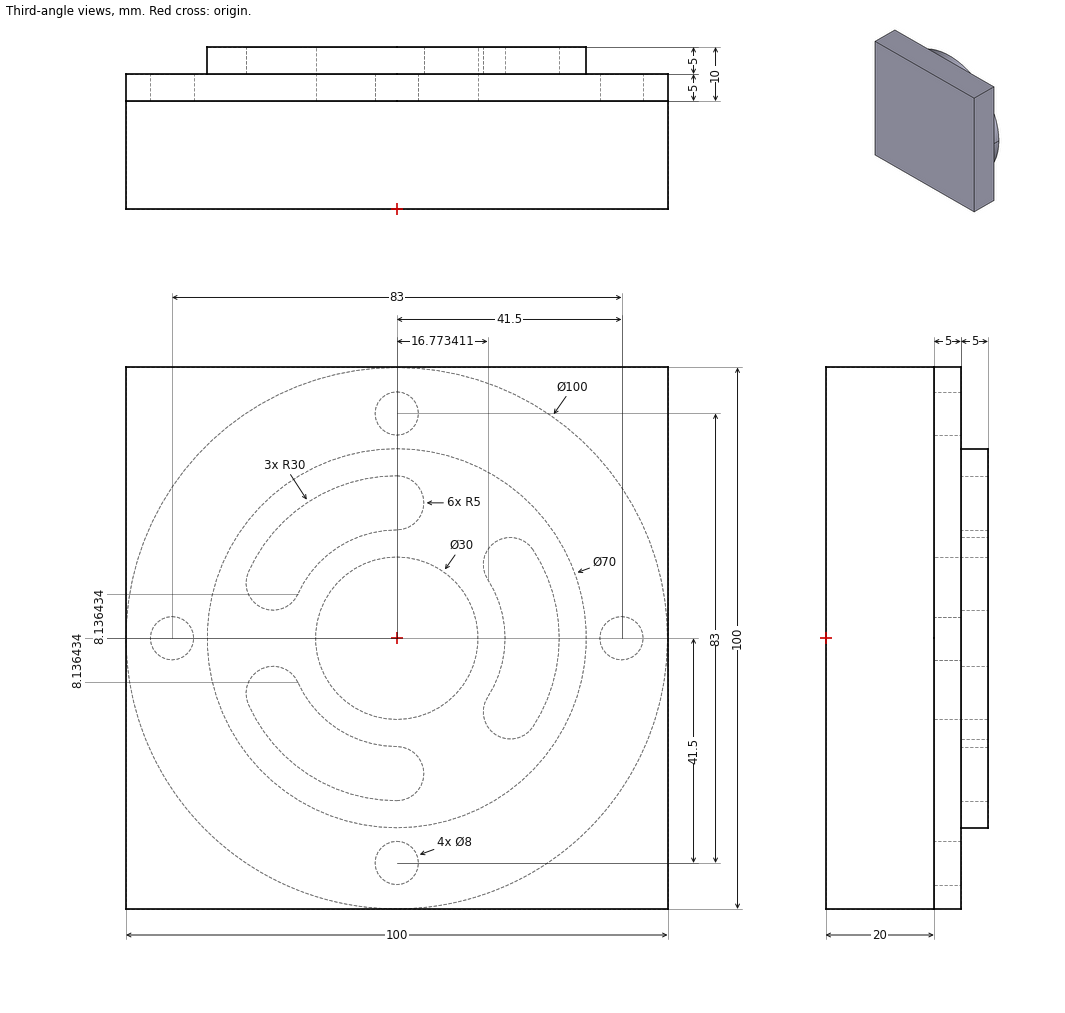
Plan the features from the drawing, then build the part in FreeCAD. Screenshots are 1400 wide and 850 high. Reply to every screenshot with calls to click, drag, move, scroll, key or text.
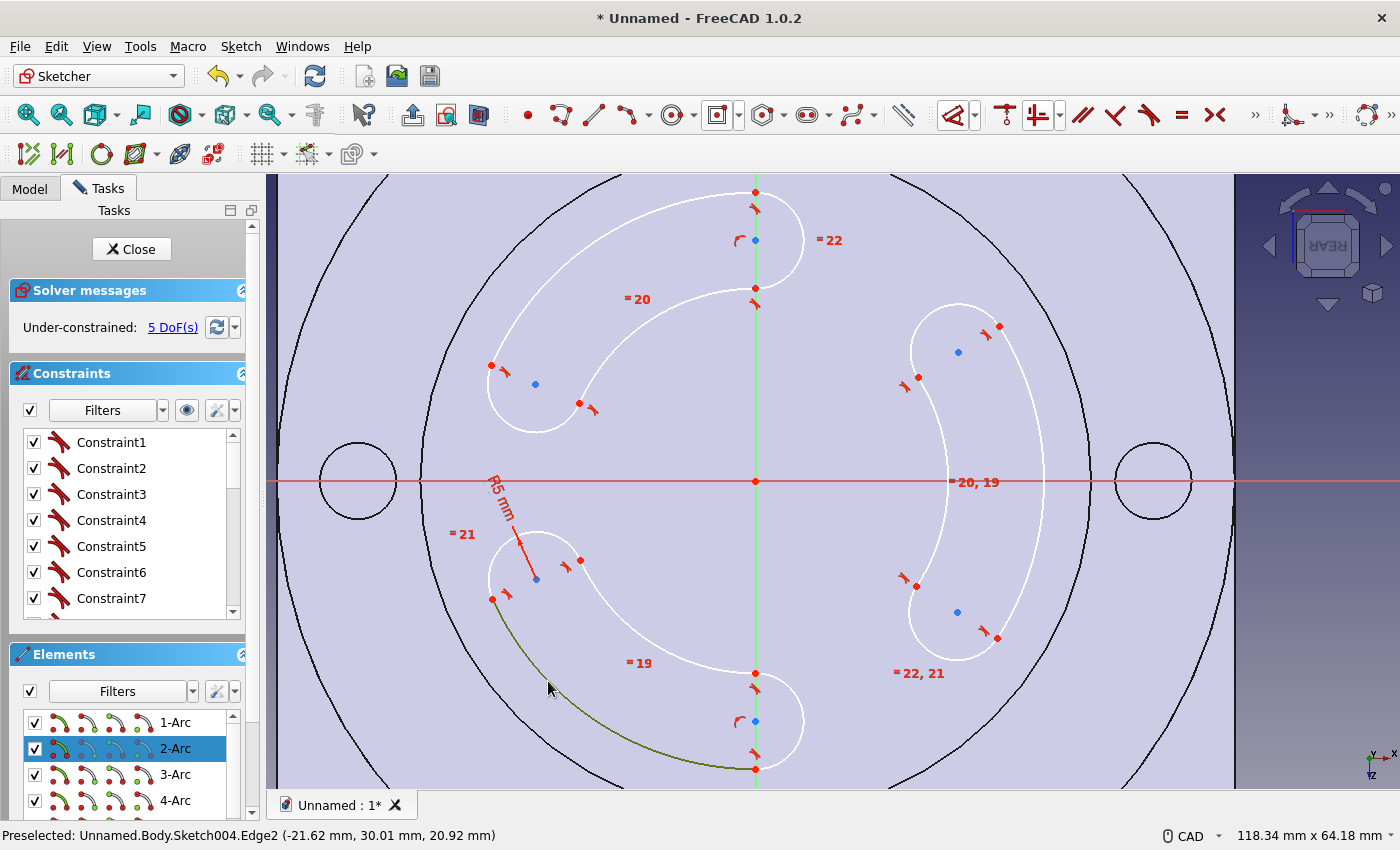
click(974, 116)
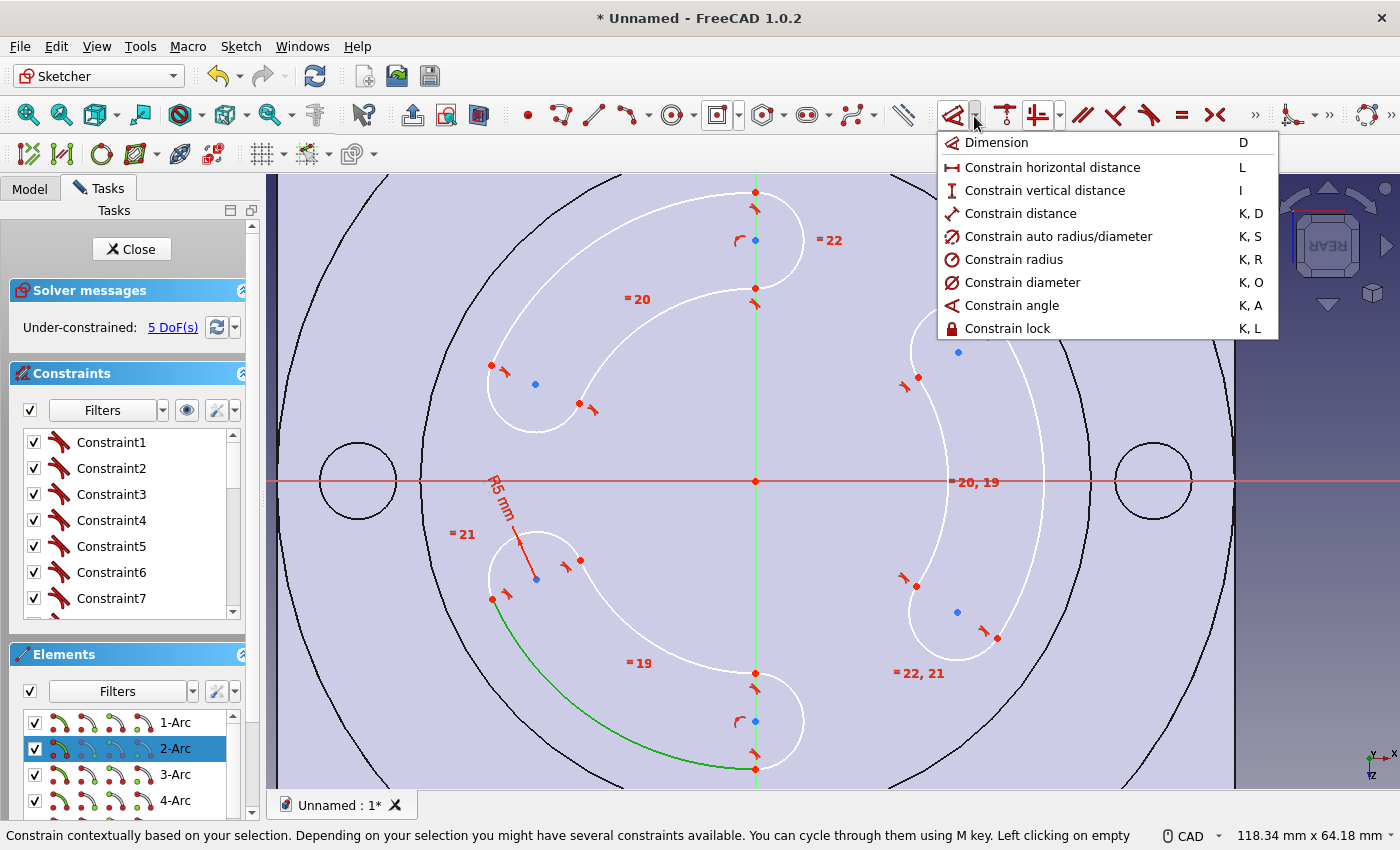
click(1108, 260)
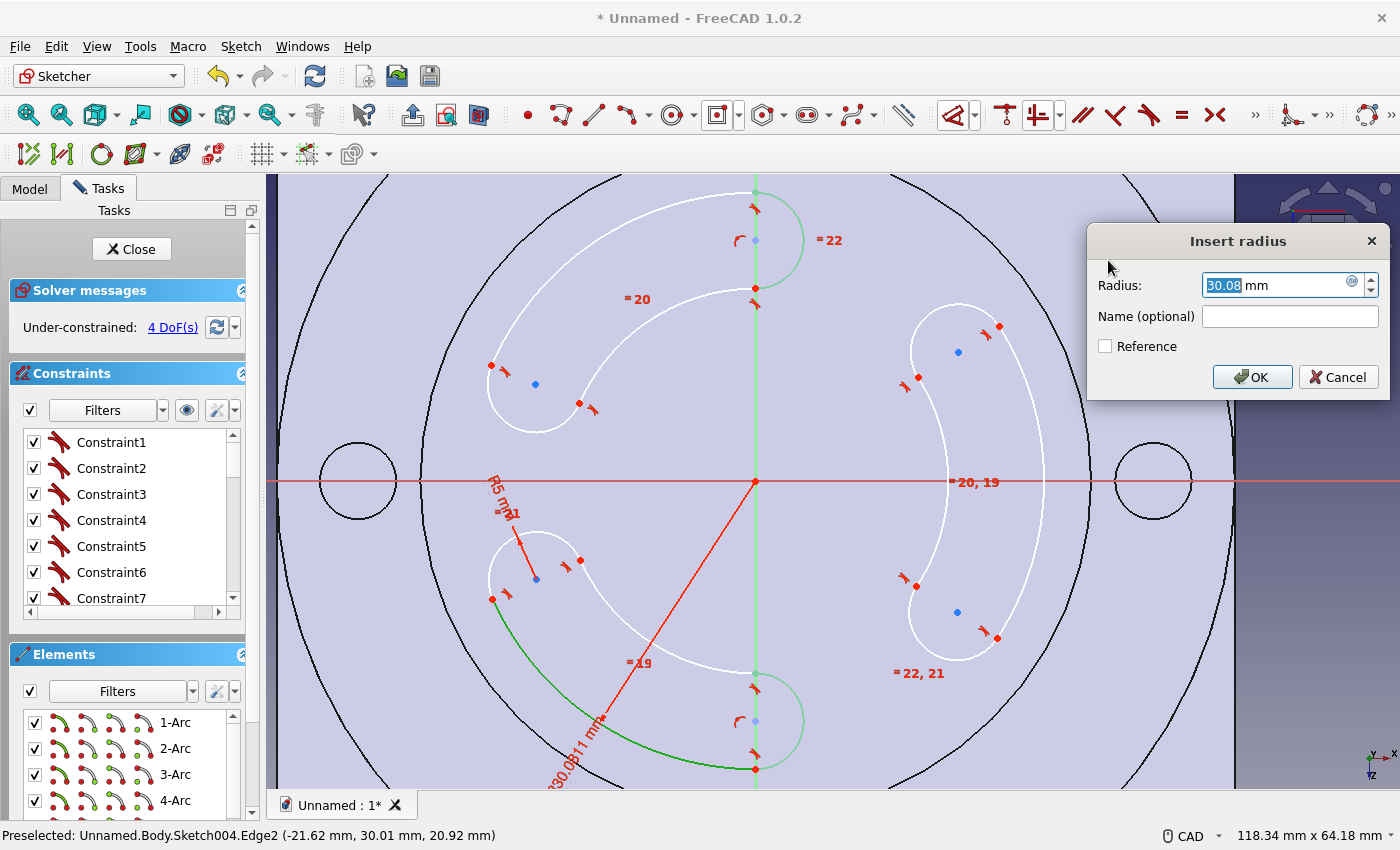
text(30)
key(Return)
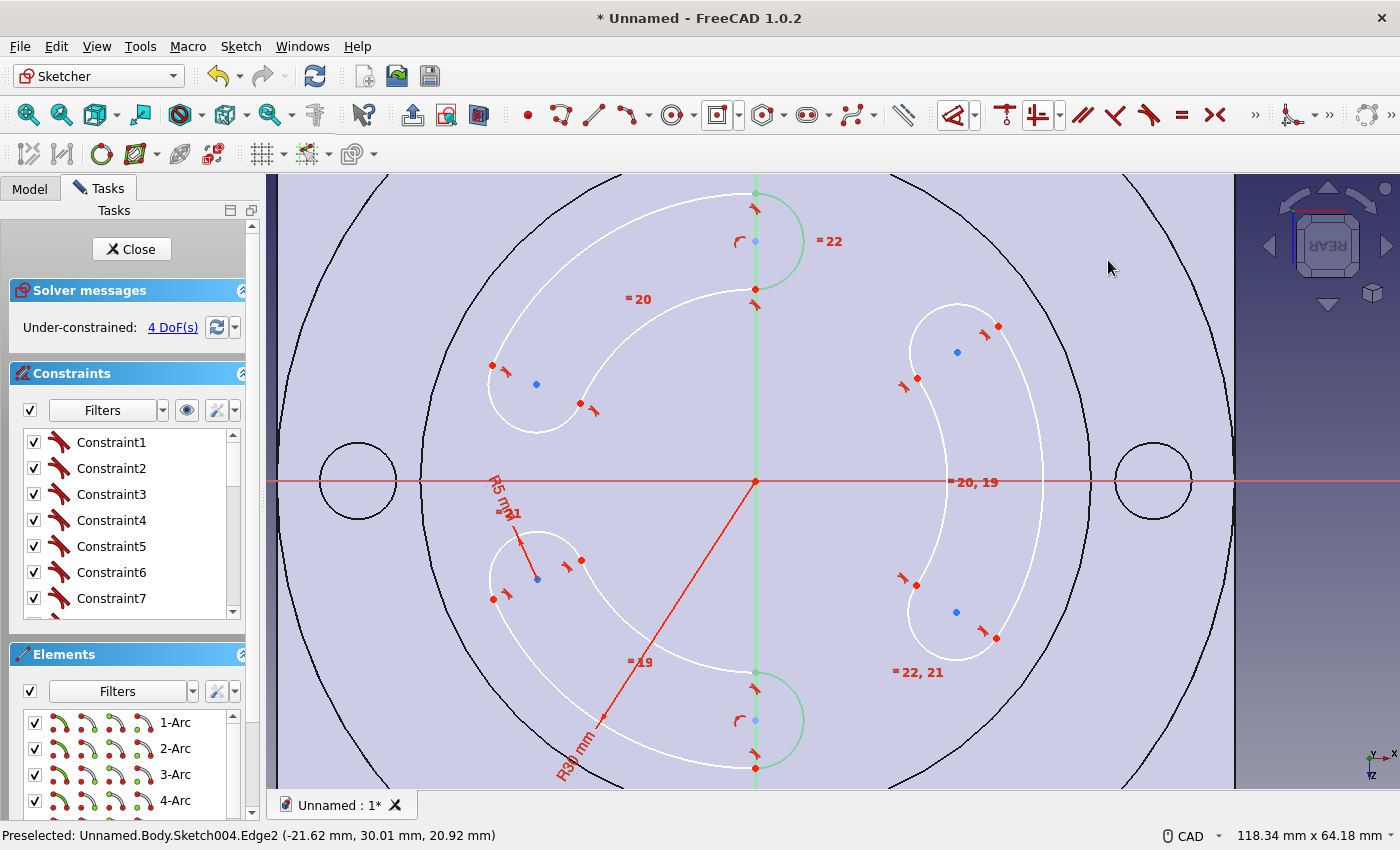
click(581, 560)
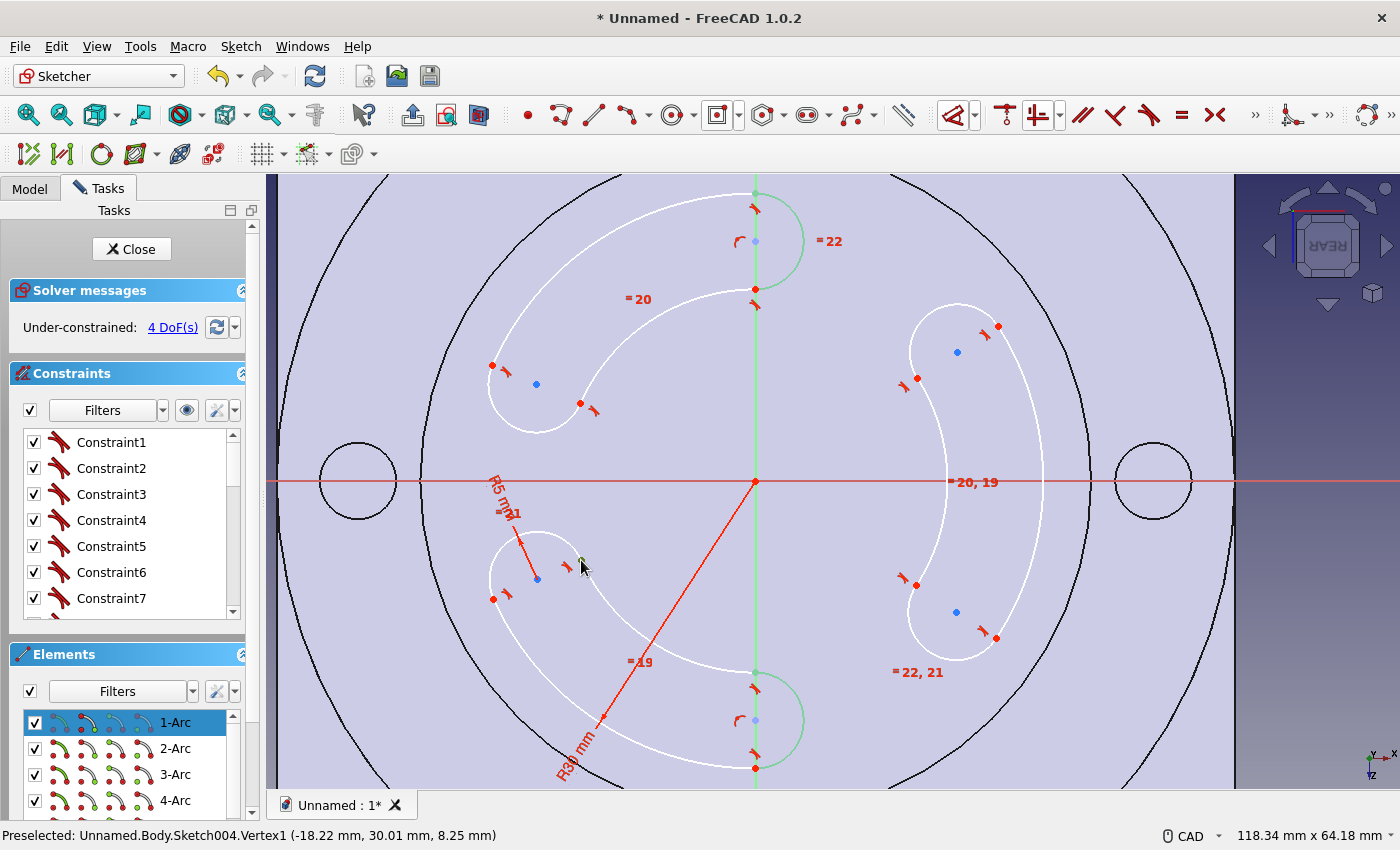
key(i)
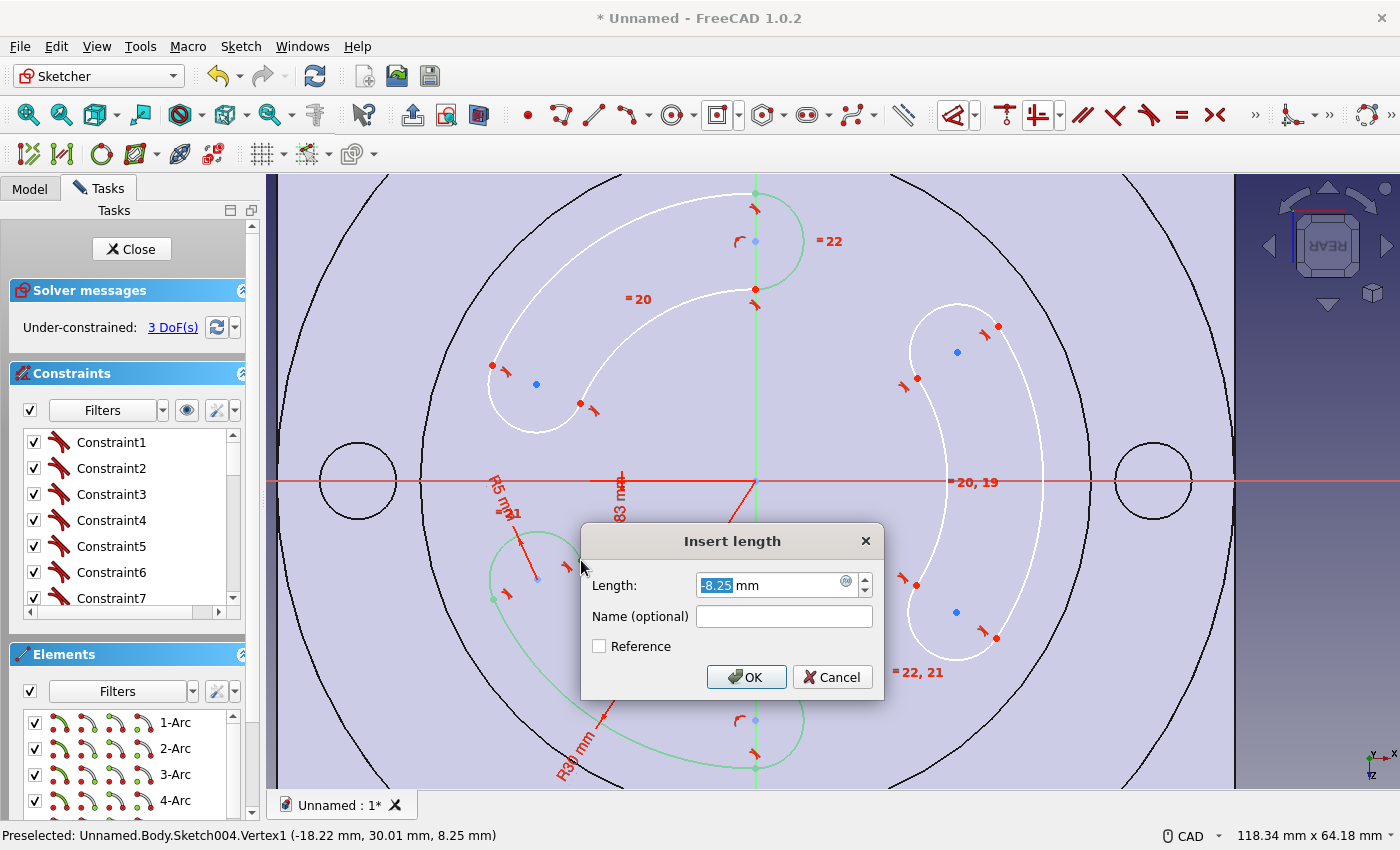
text(-8.136434)
key(Return)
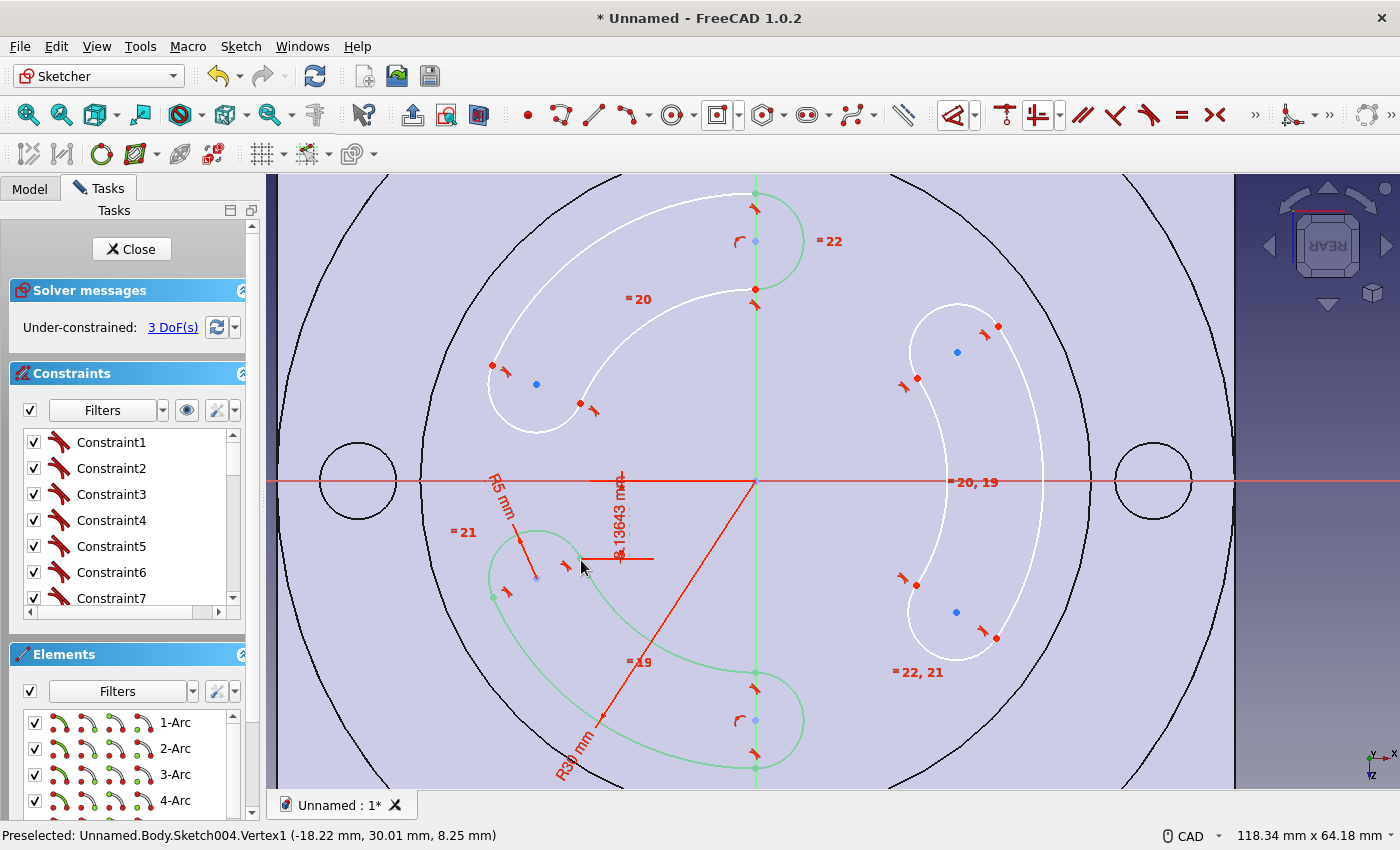
click(580, 404)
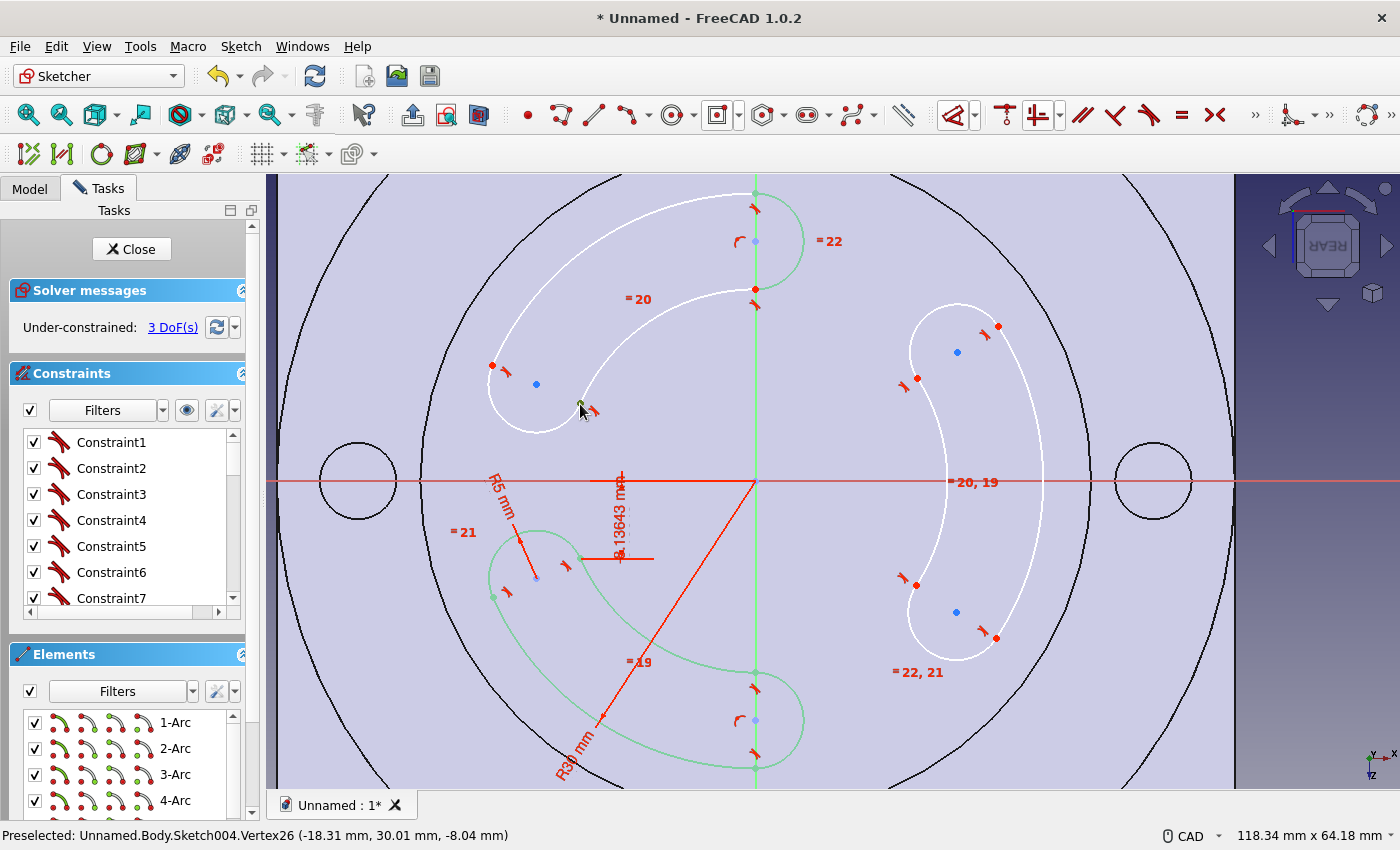
key(i)